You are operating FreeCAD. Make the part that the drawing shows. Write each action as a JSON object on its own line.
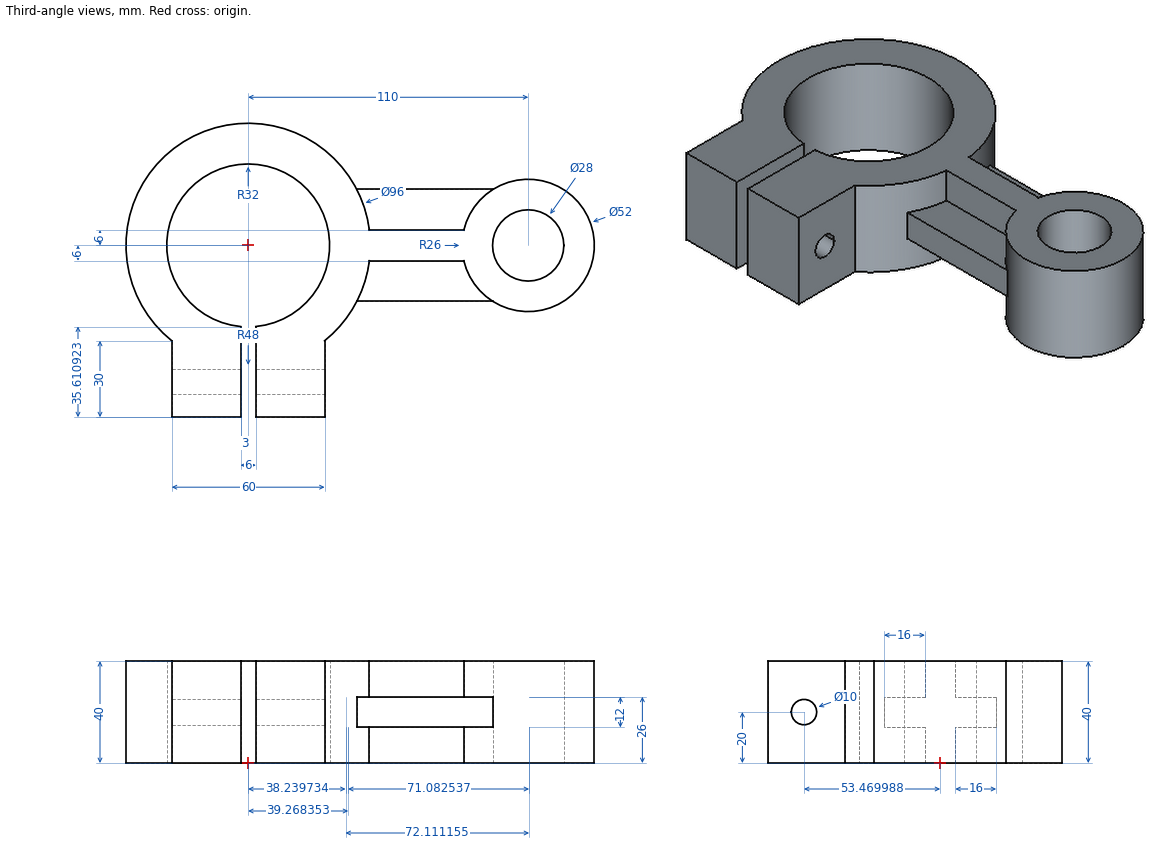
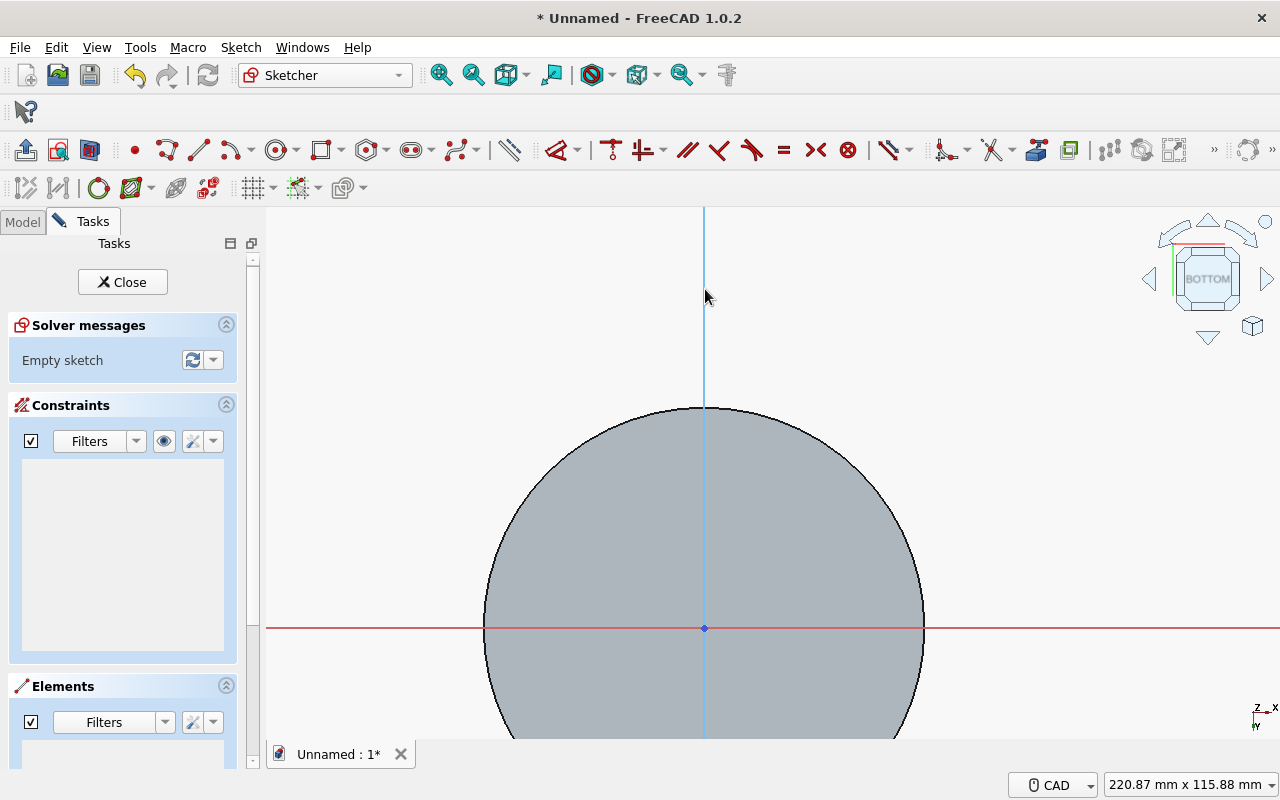
{"action": "left_click", "coordinate": [168, 150]}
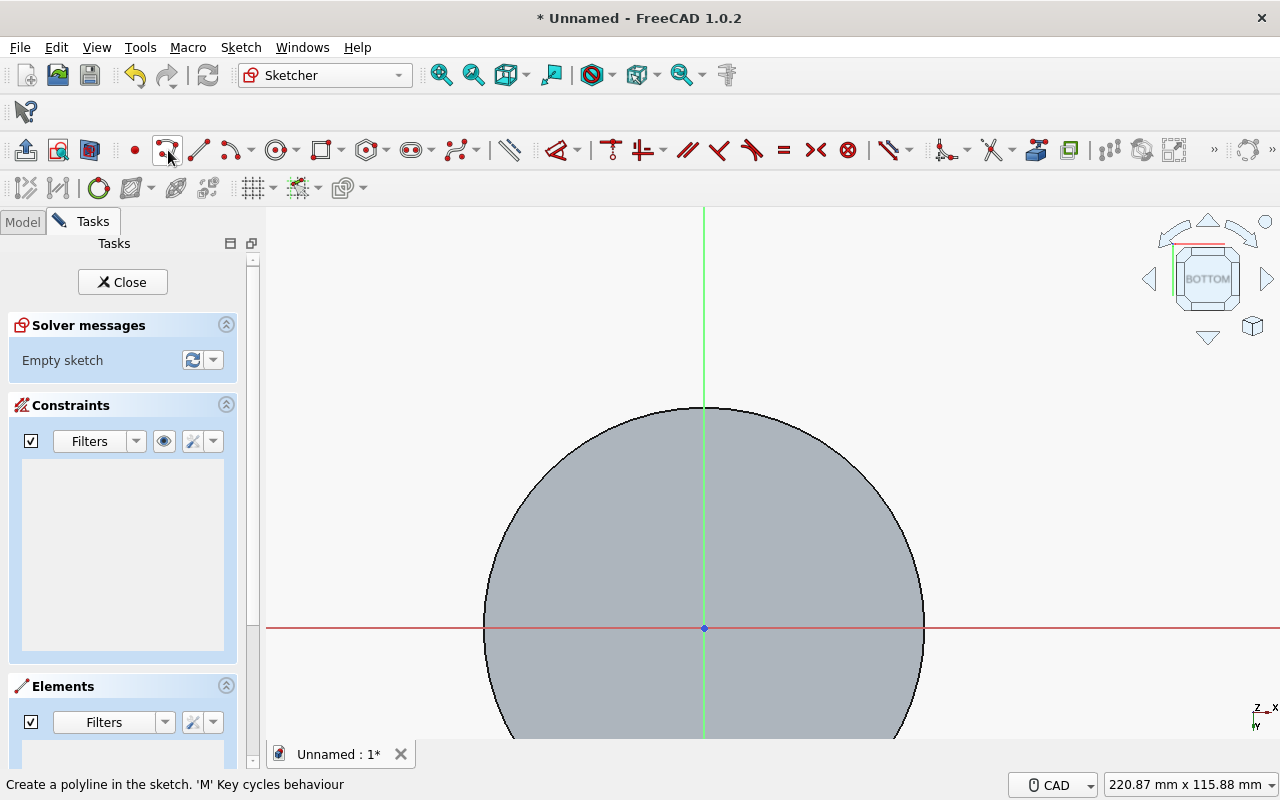
{"action": "left_click", "coordinate": [566, 456]}
{"action": "left_click", "coordinate": [566, 318]}
{"action": "left_click", "coordinate": [842, 318]}
{"action": "left_click", "coordinate": [842, 456]}
{"action": "right_click", "coordinate": [842, 456]}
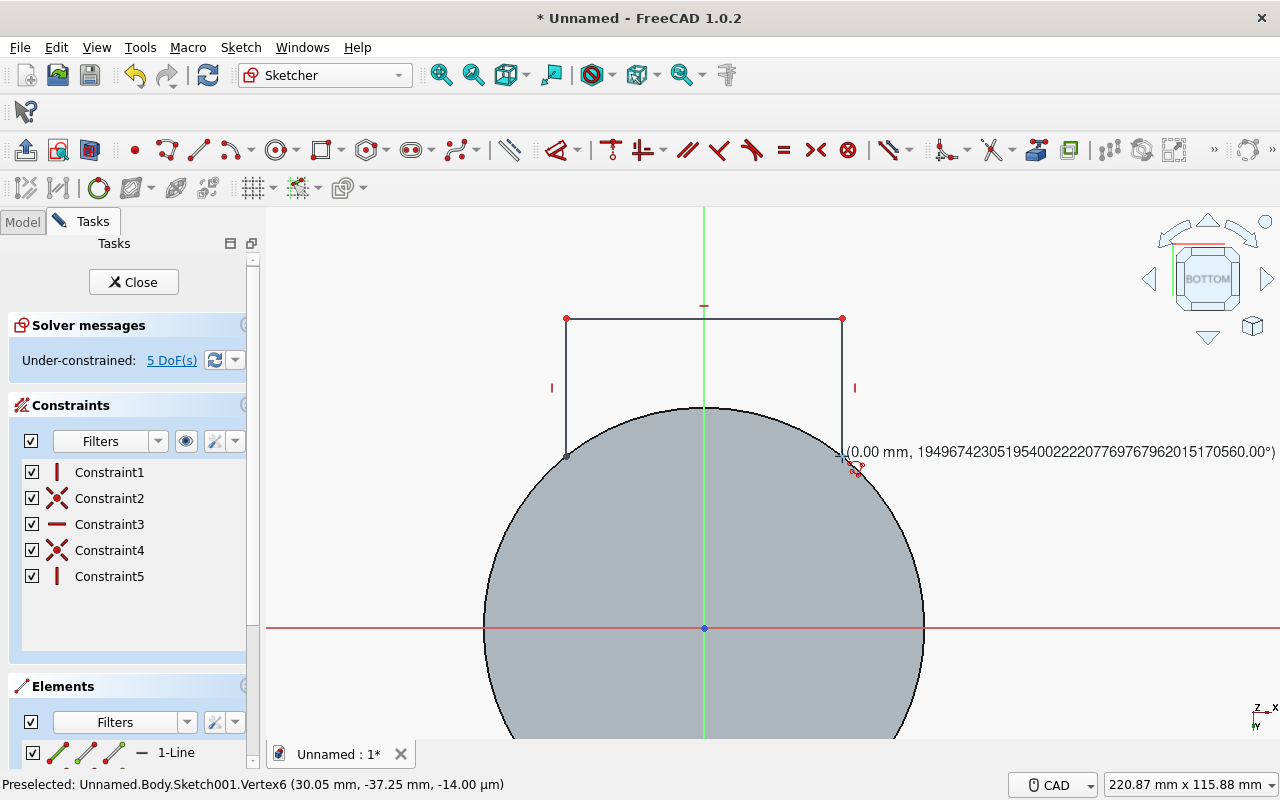
{"action": "left_click", "coordinate": [254, 150]}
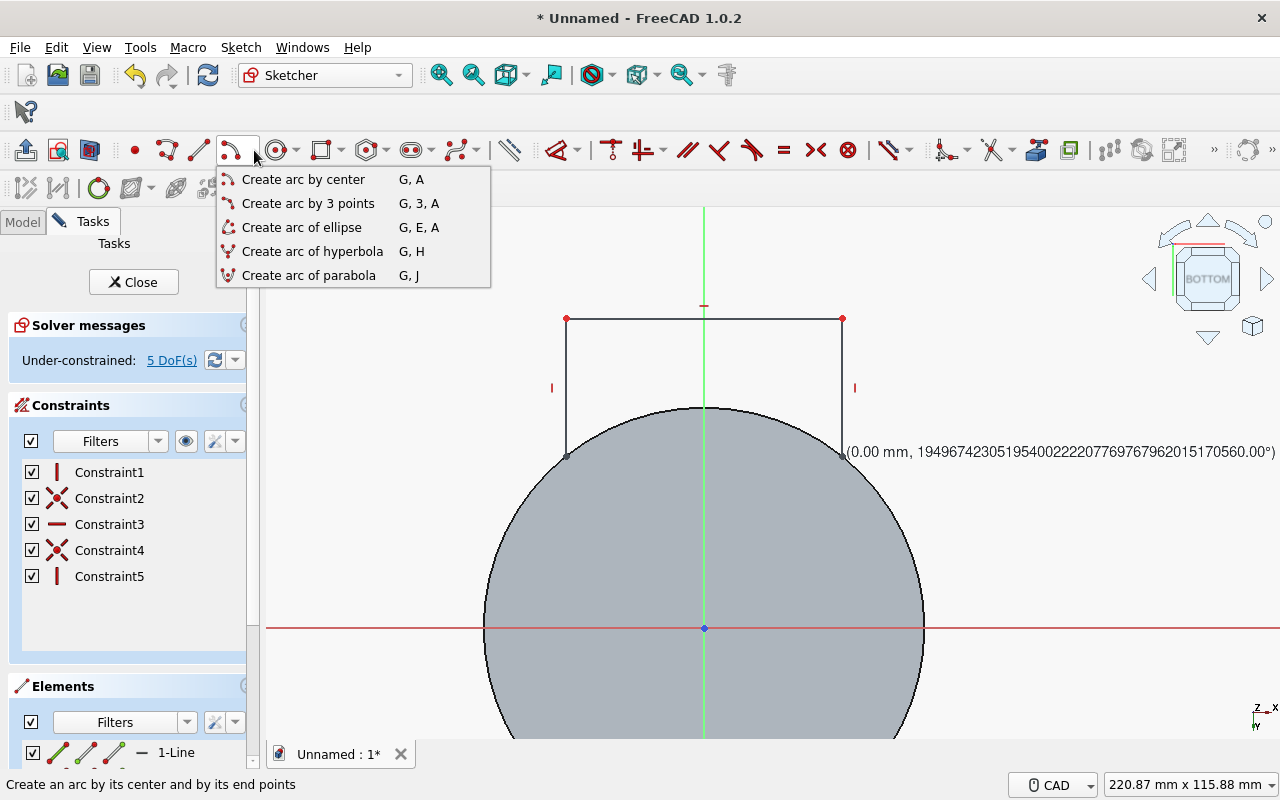
{"action": "left_click", "coordinate": [354, 203]}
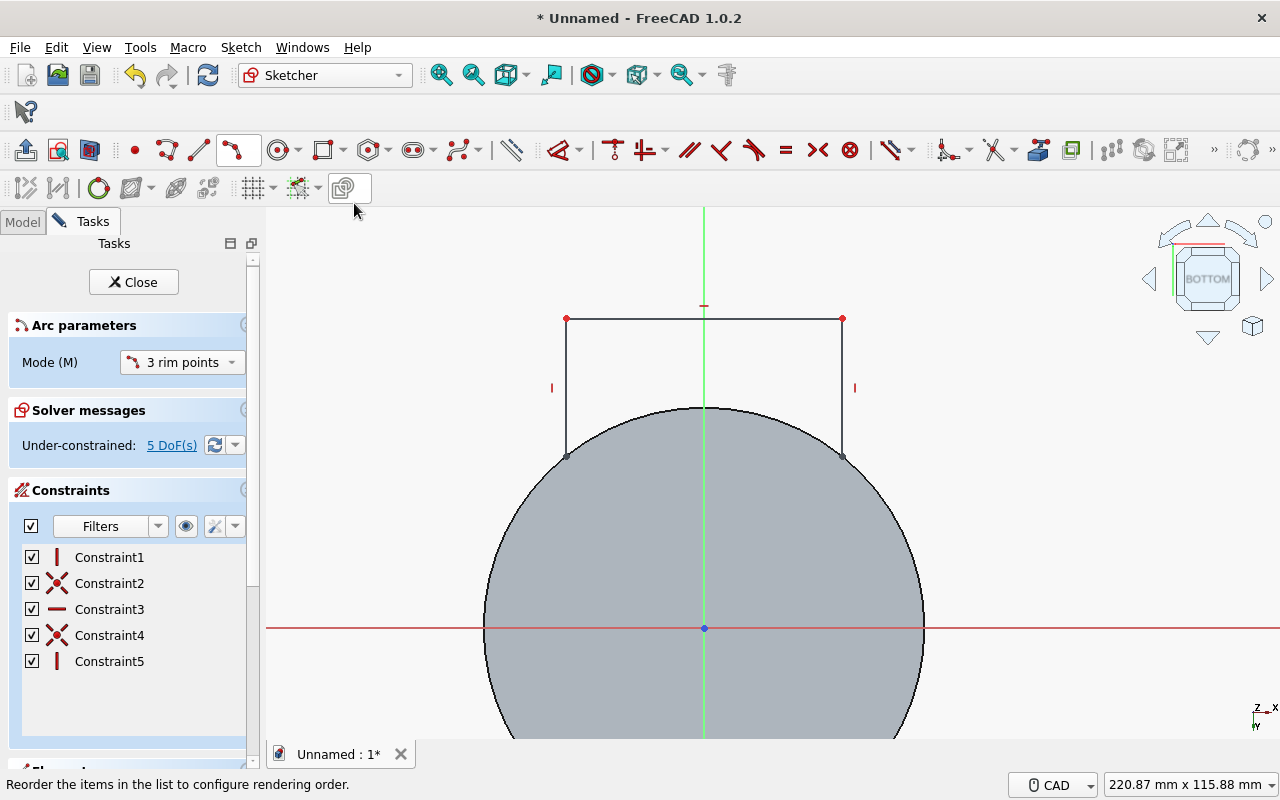
{"action": "left_click", "coordinate": [842, 457]}
{"action": "left_click", "coordinate": [566, 457]}
{"action": "left_click", "coordinate": [734, 410]}
{"action": "key", "text": "Escape"}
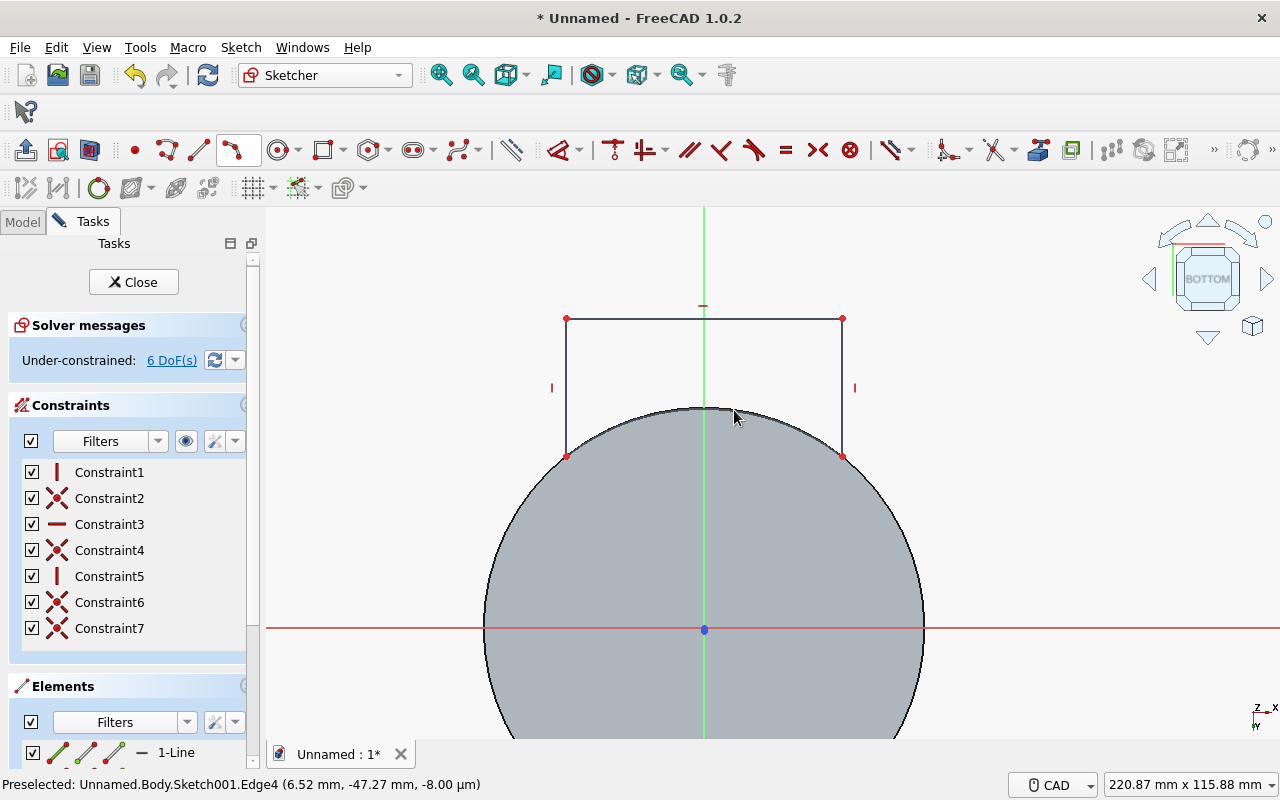
{"action": "left_click_drag", "start_coordinate": [694, 618], "coordinate": [714, 641]}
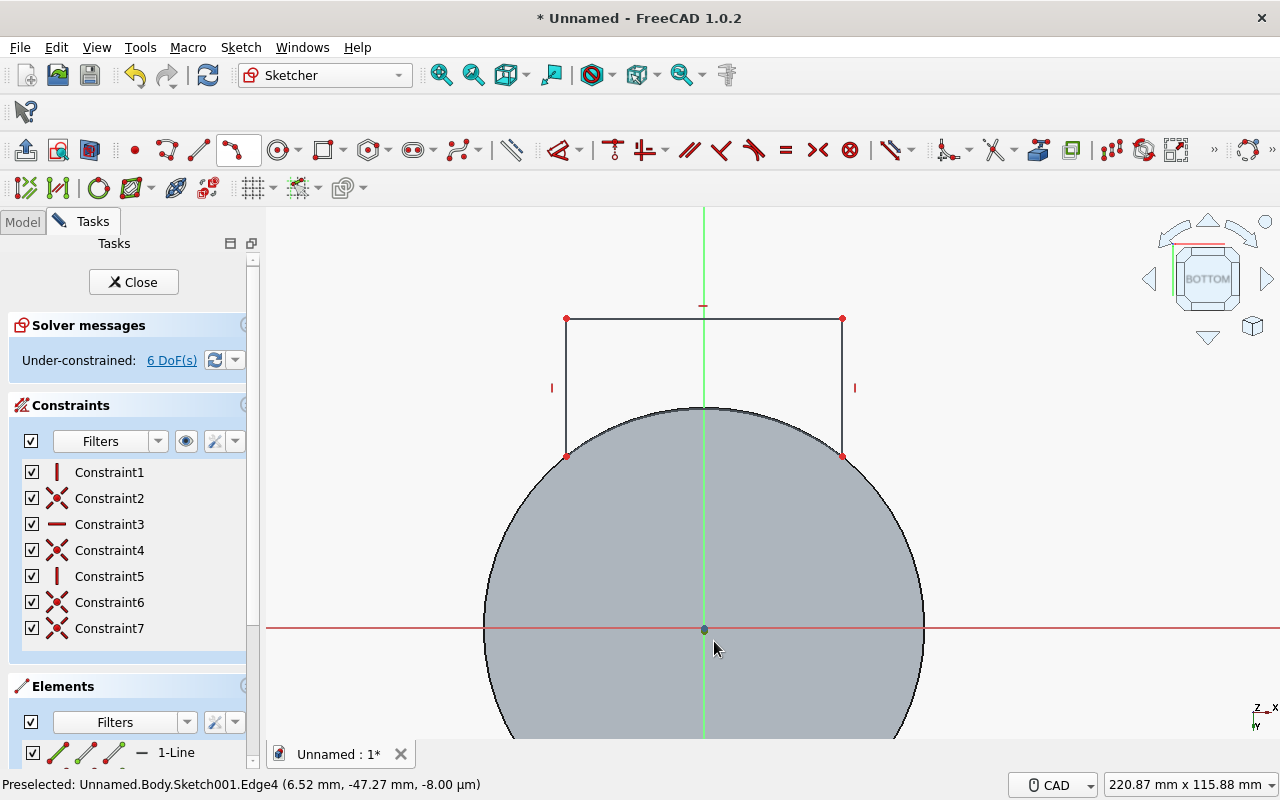
{"action": "left_click", "coordinate": [614, 150]}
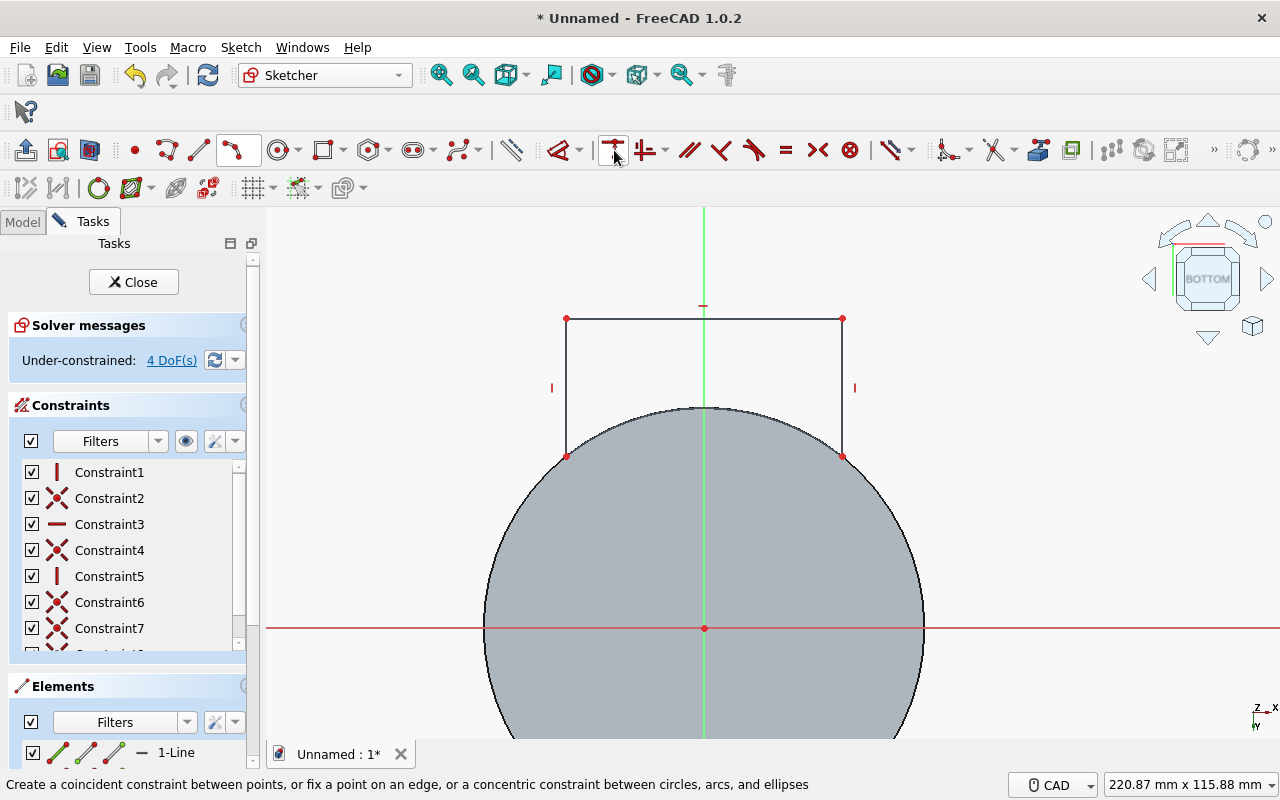
{"action": "left_click", "coordinate": [558, 150]}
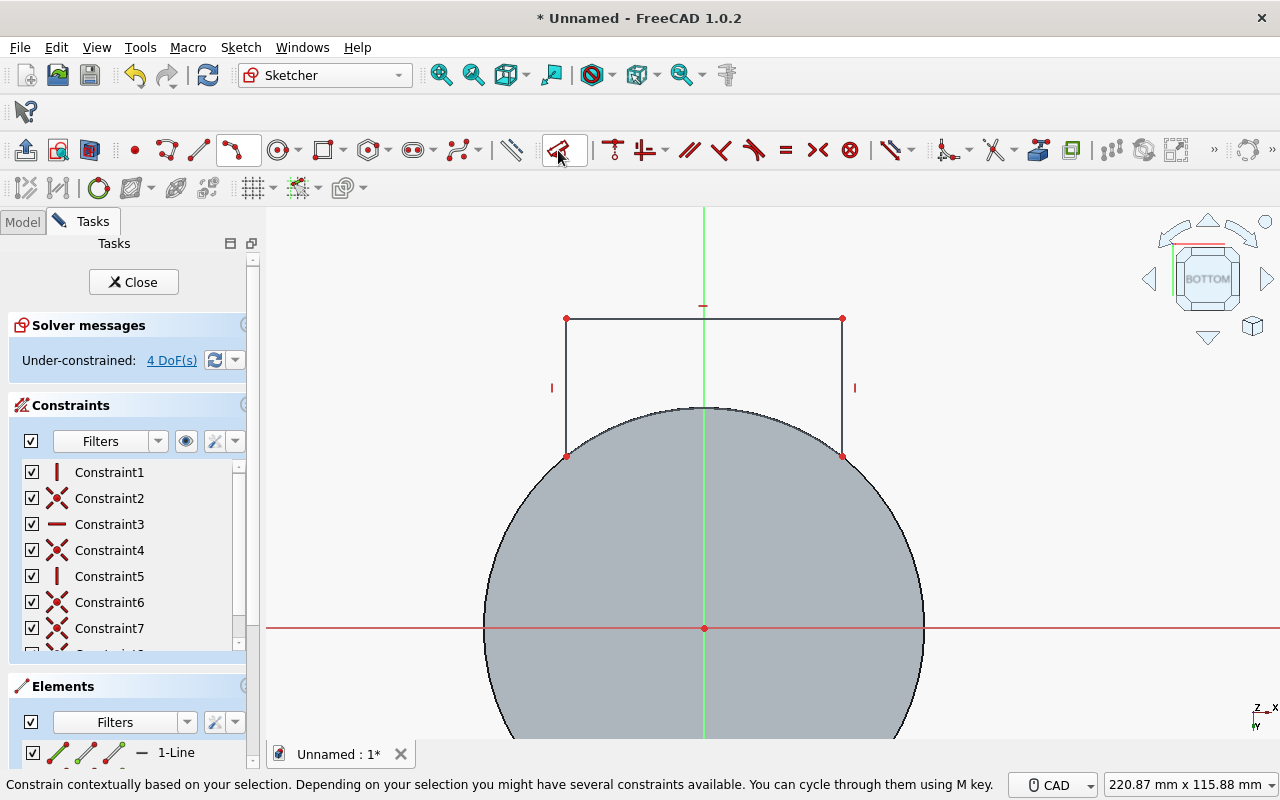
{"action": "left_click", "coordinate": [763, 416]}
{"action": "left_click", "coordinate": [772, 385]}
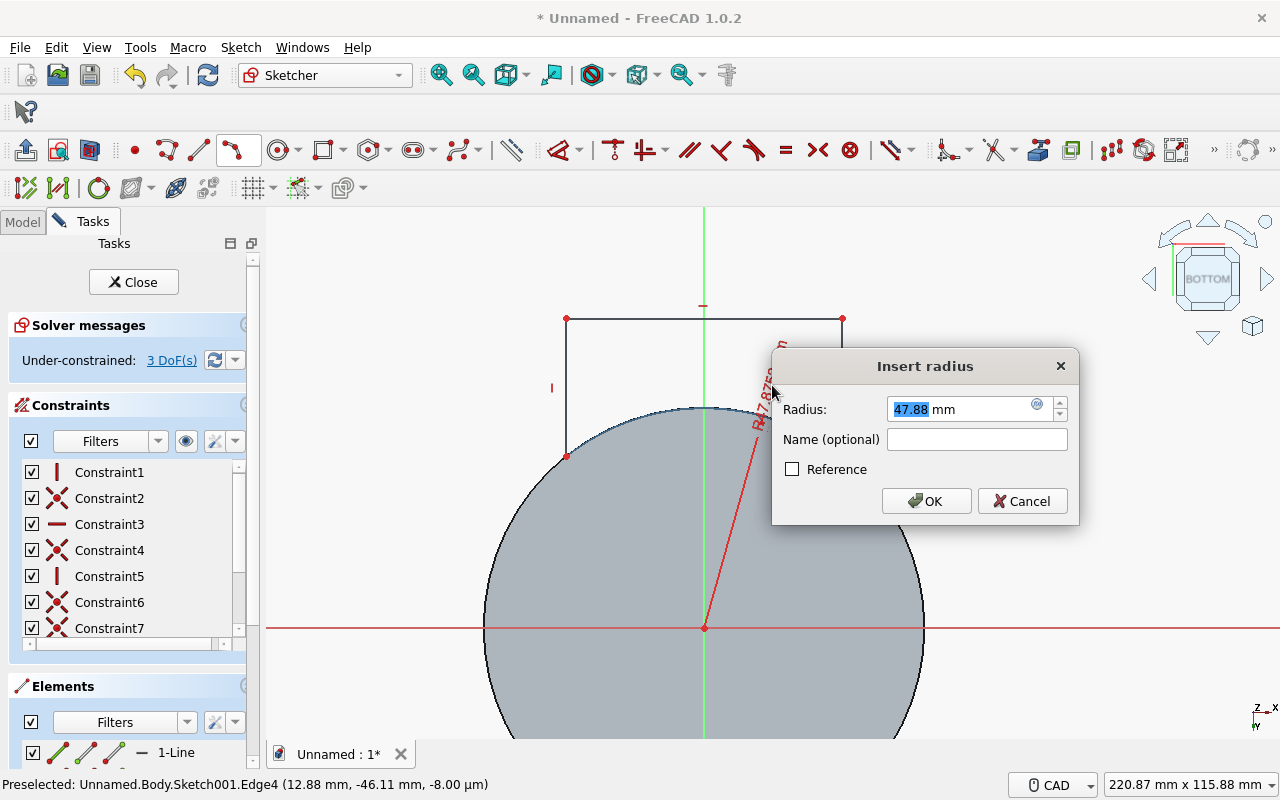
{"action": "type", "text": "48"}
{"action": "key", "text": "Return"}